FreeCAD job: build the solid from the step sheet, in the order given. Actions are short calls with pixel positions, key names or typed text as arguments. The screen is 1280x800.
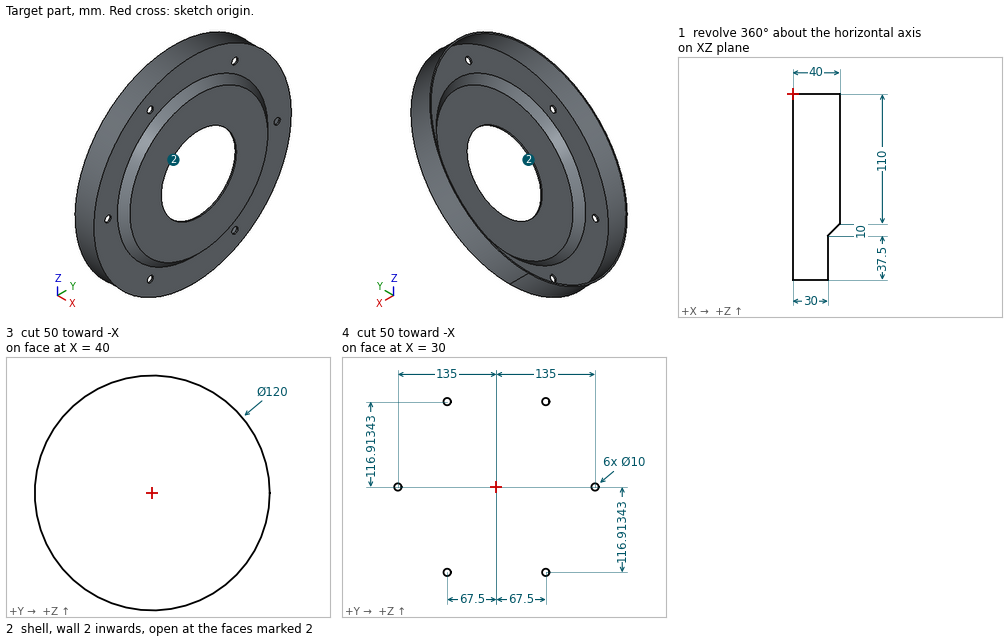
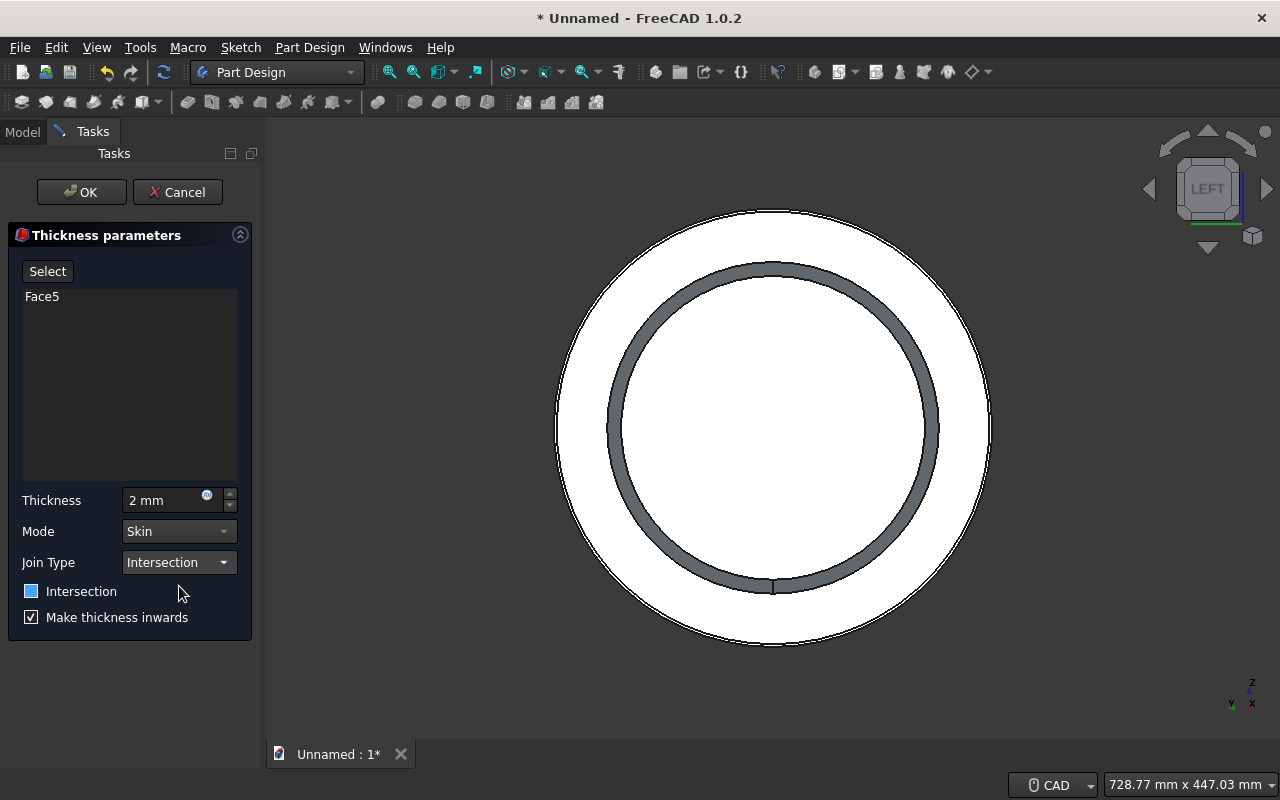
click(82, 192)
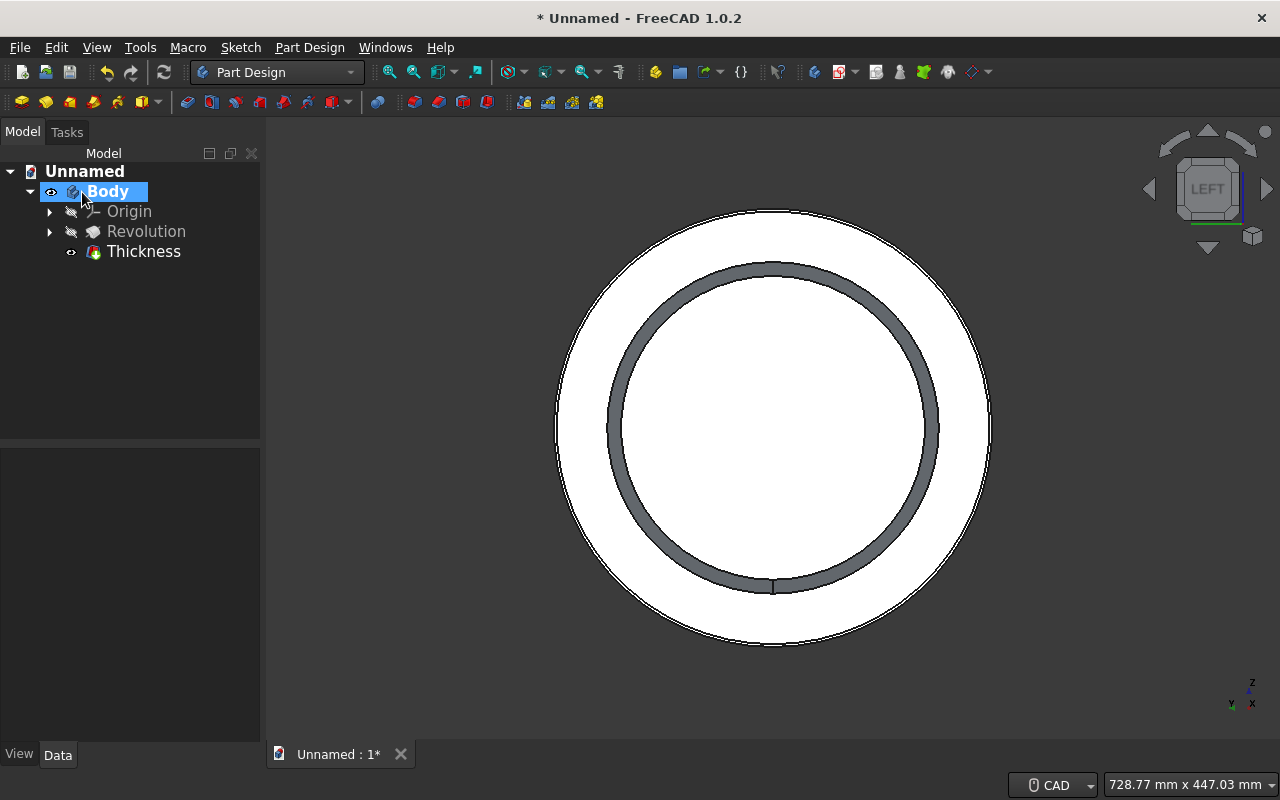
key(0)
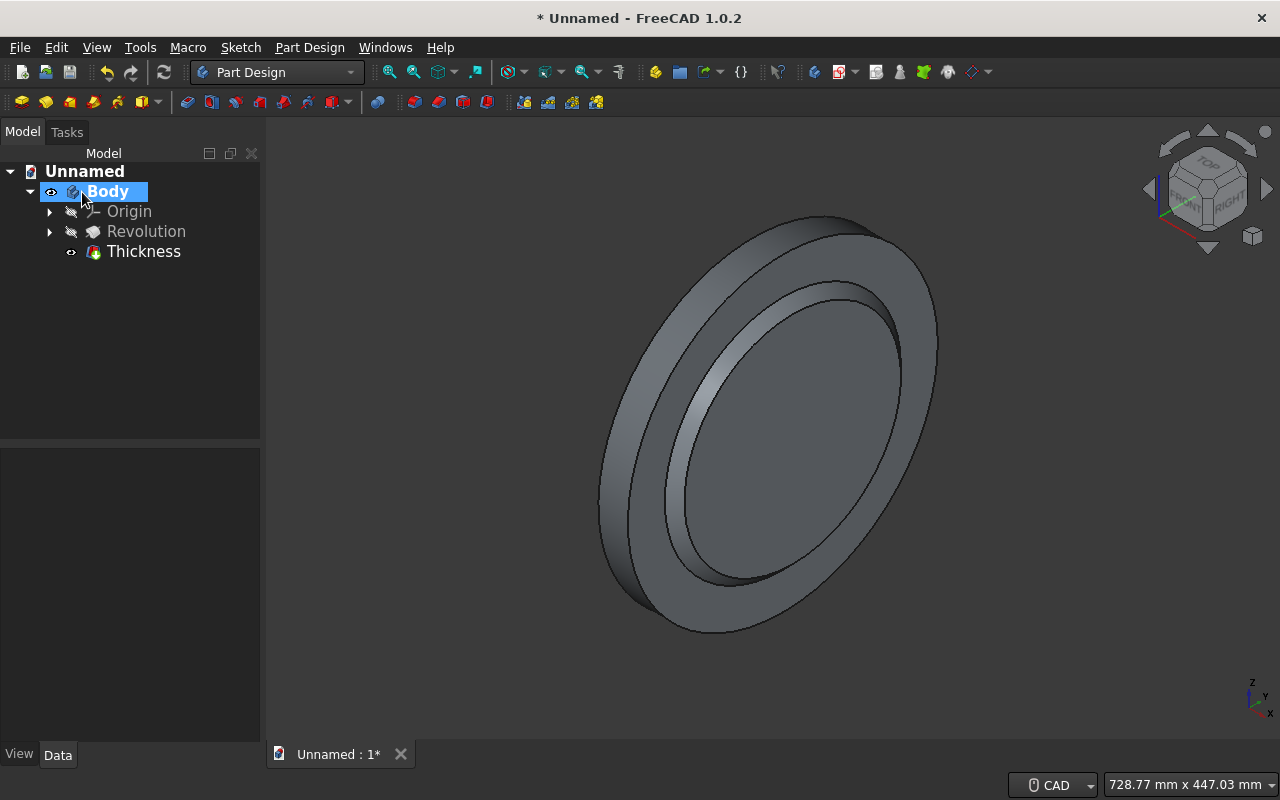
click(793, 438)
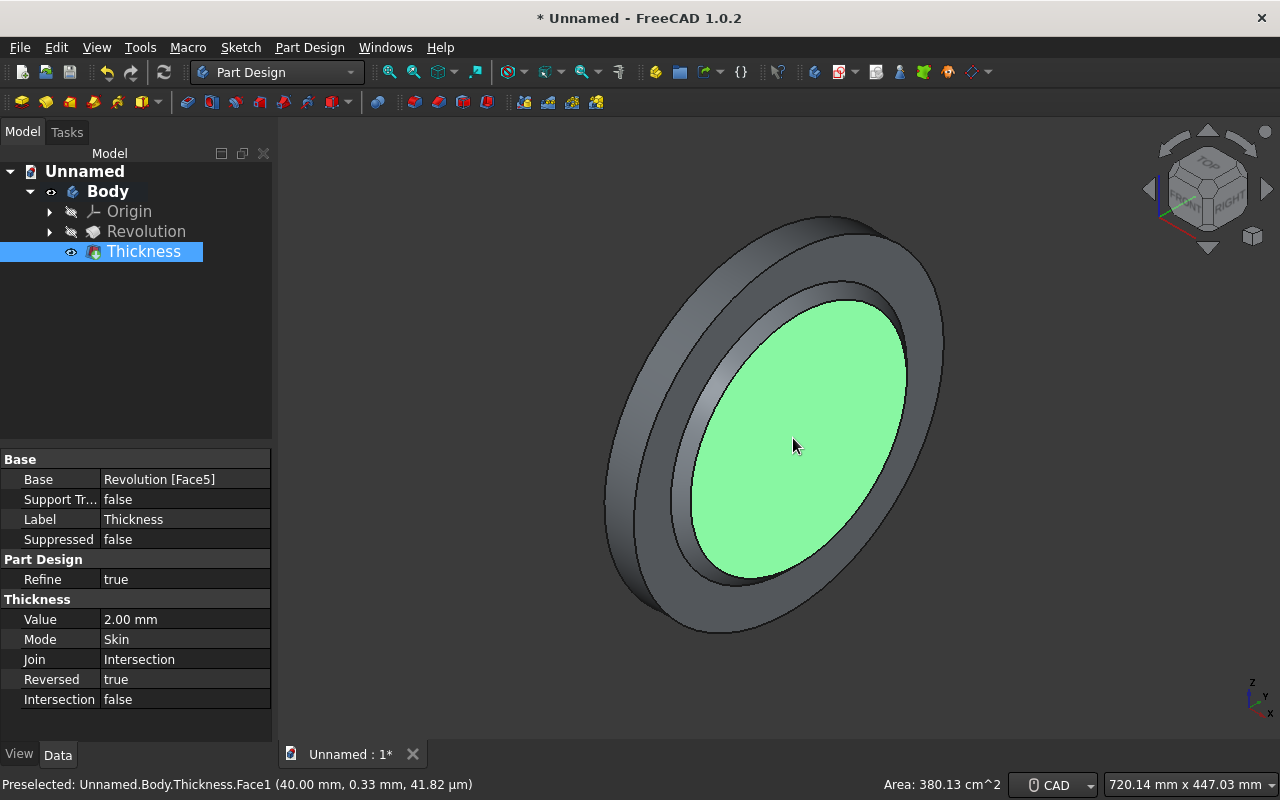
click(840, 72)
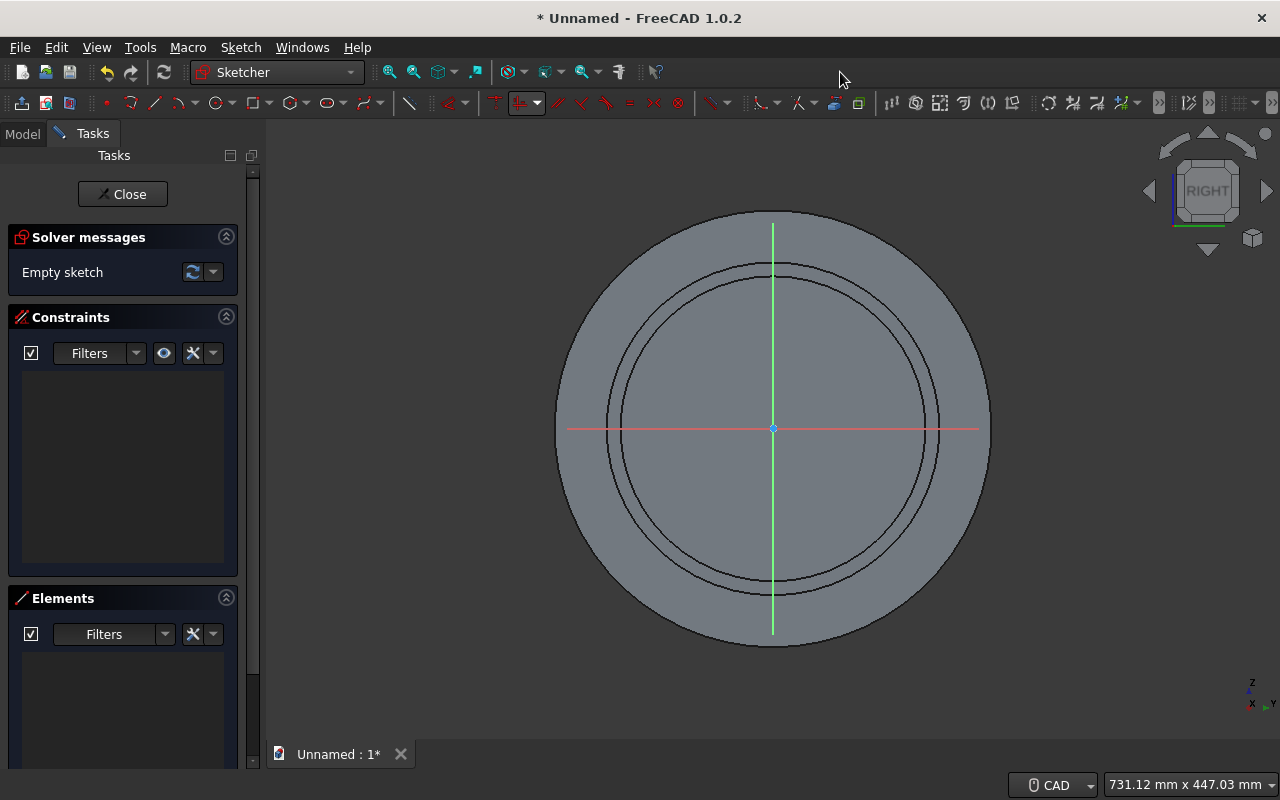
scroll(829, 429, up, 4)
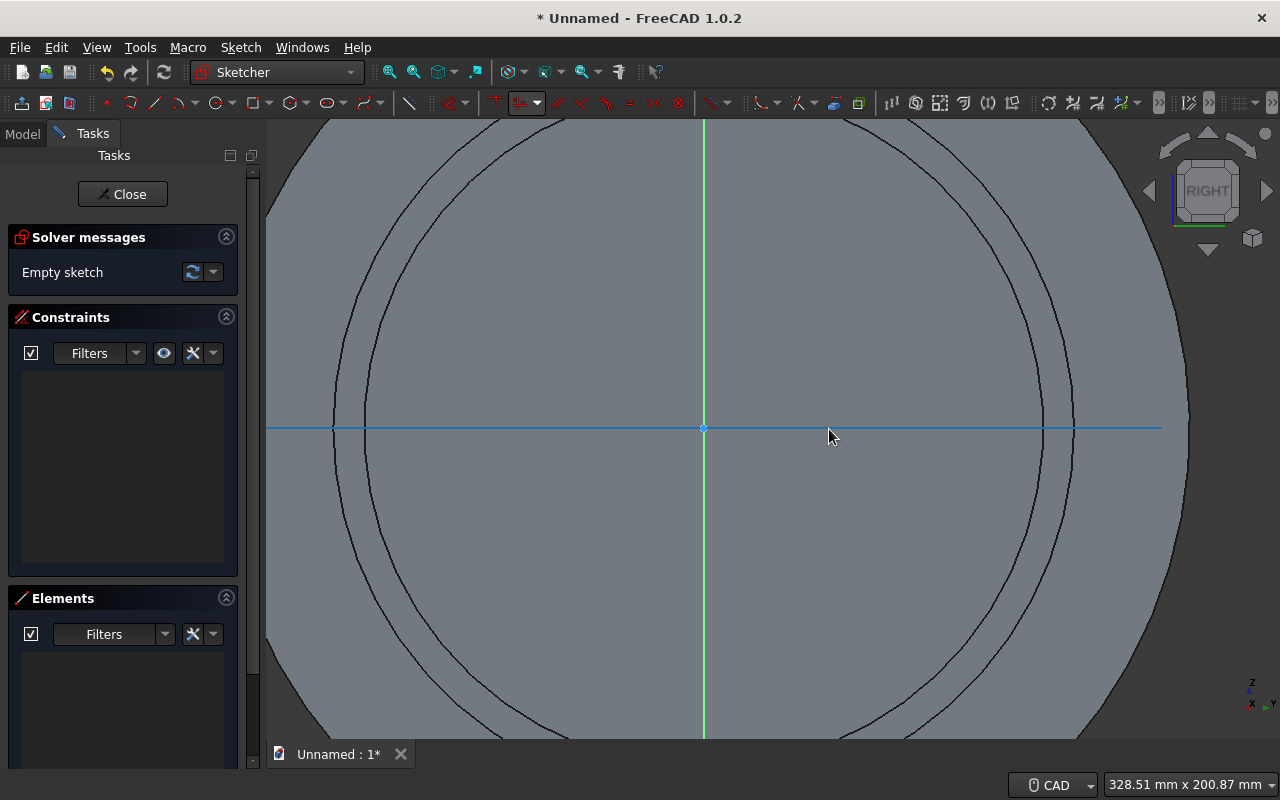
click(216, 104)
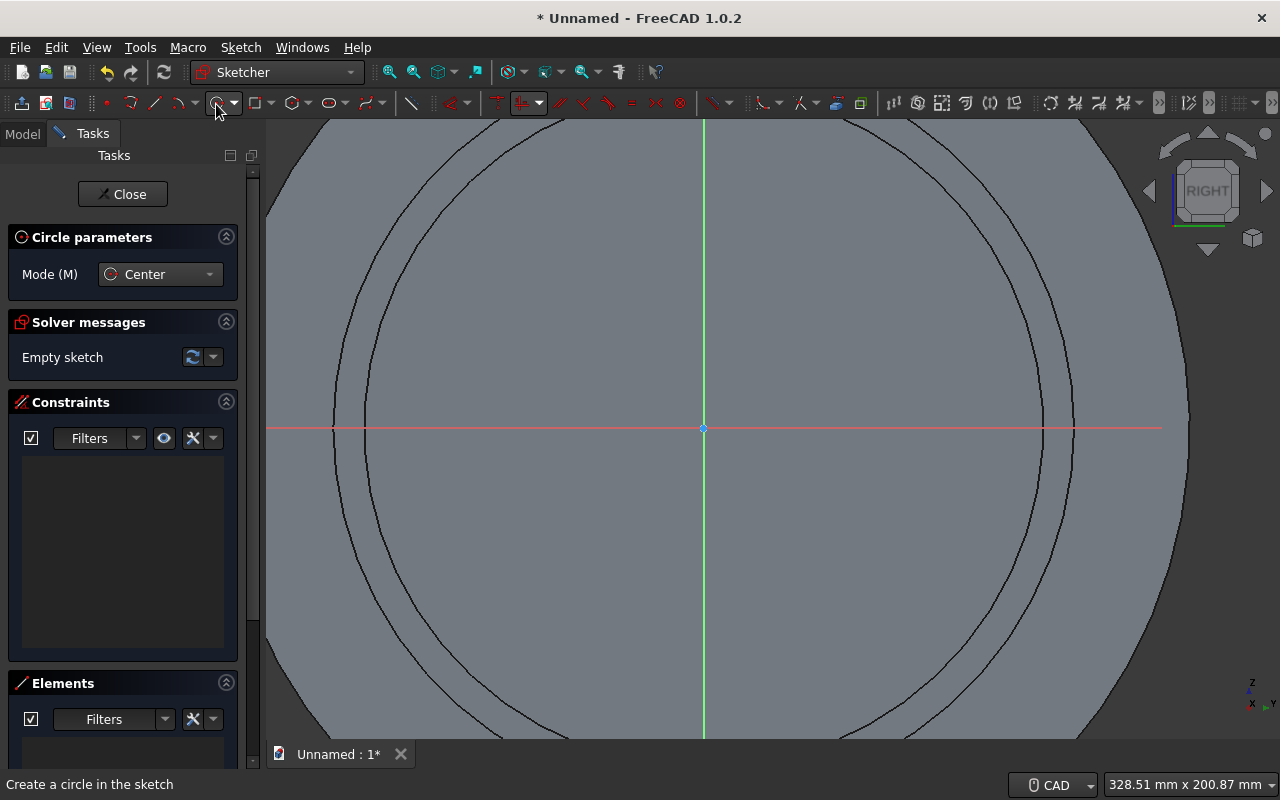
click(704, 428)
move(835, 297)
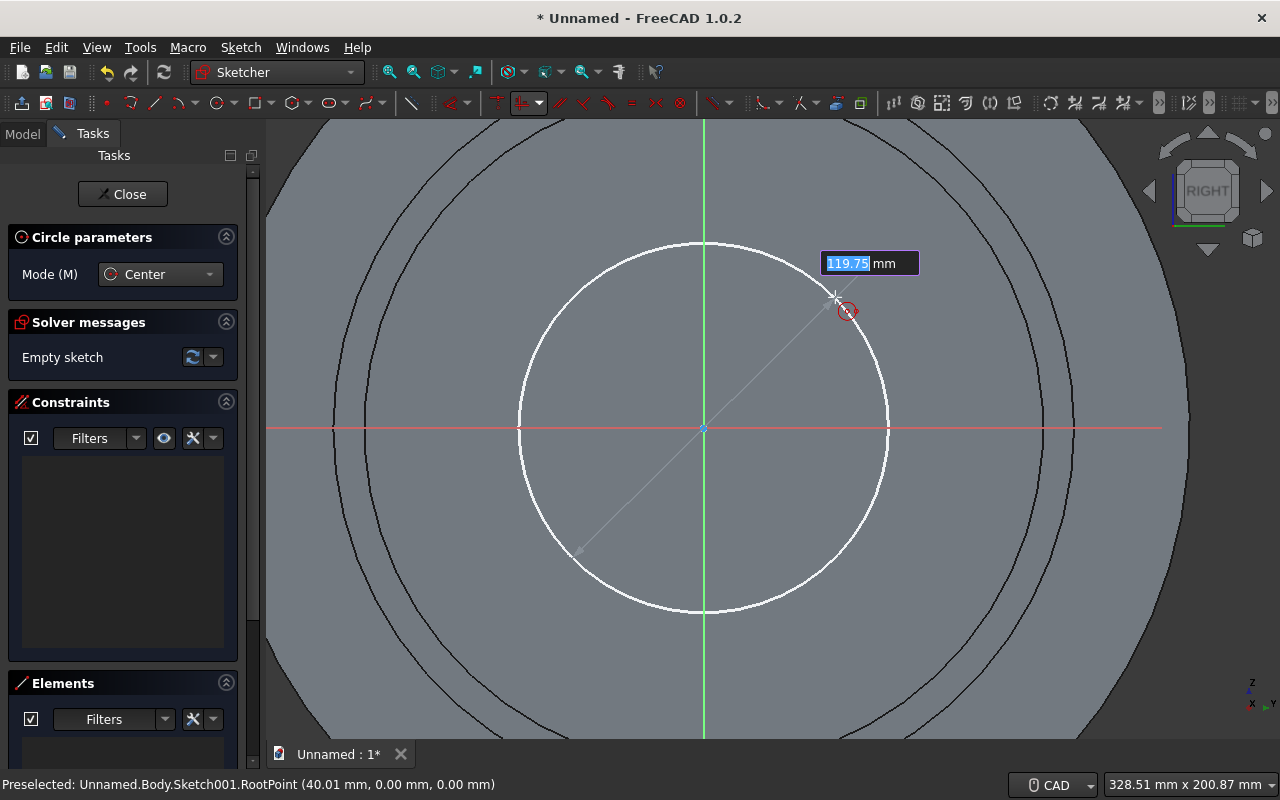
text(120)
key(Return)
key(Escape)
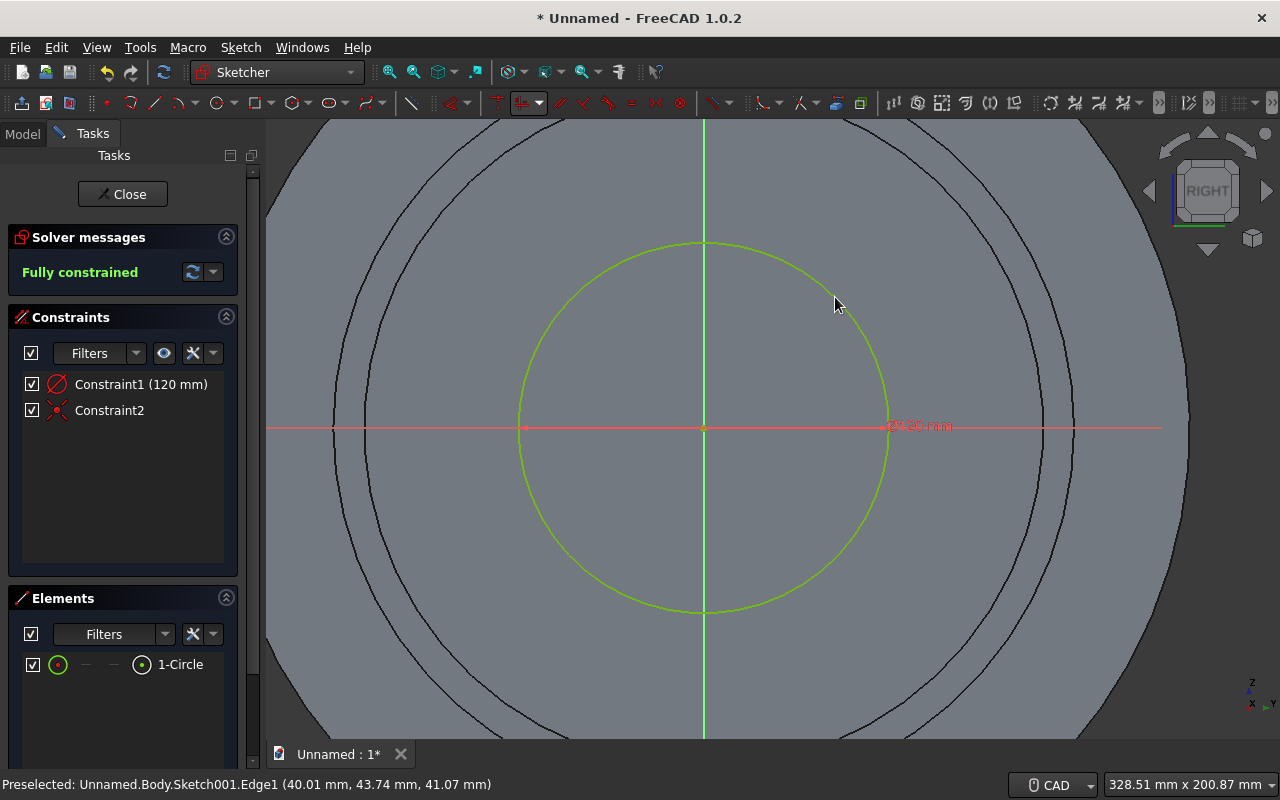
click(123, 194)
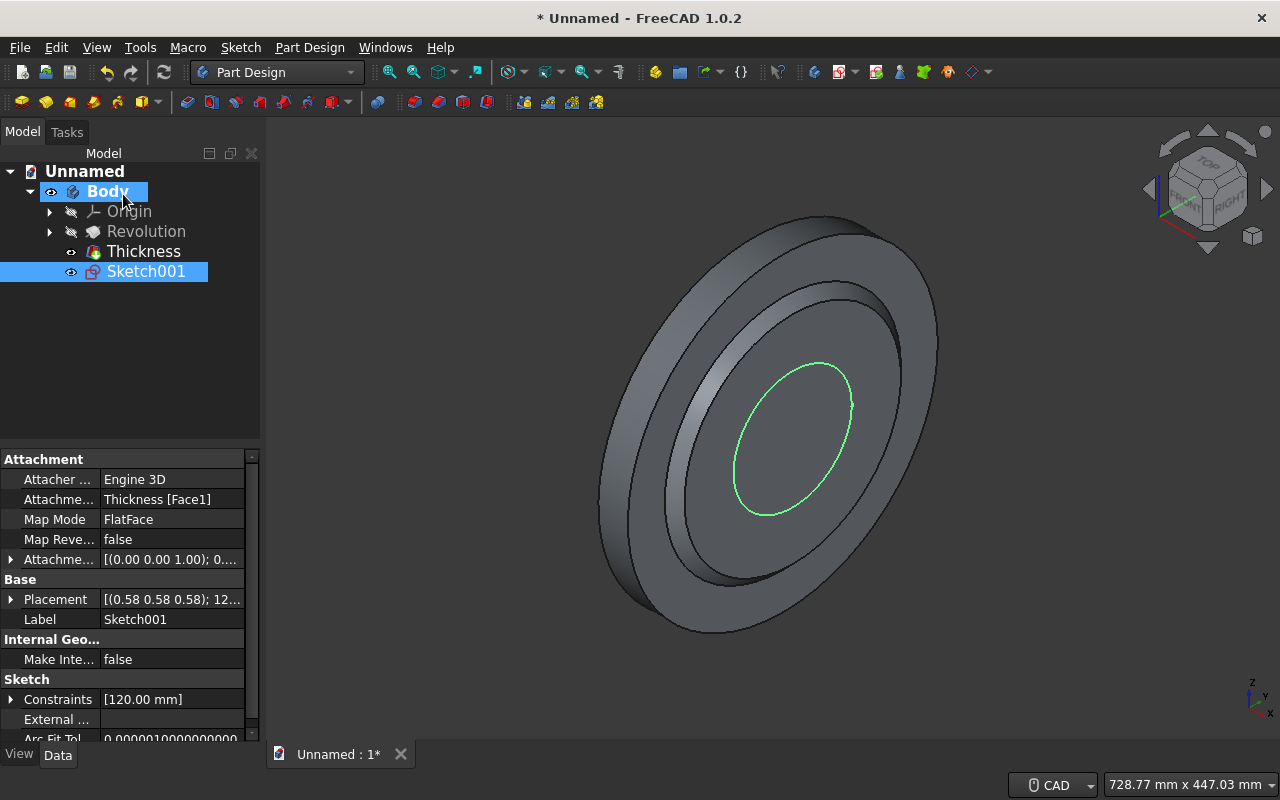
click(188, 102)